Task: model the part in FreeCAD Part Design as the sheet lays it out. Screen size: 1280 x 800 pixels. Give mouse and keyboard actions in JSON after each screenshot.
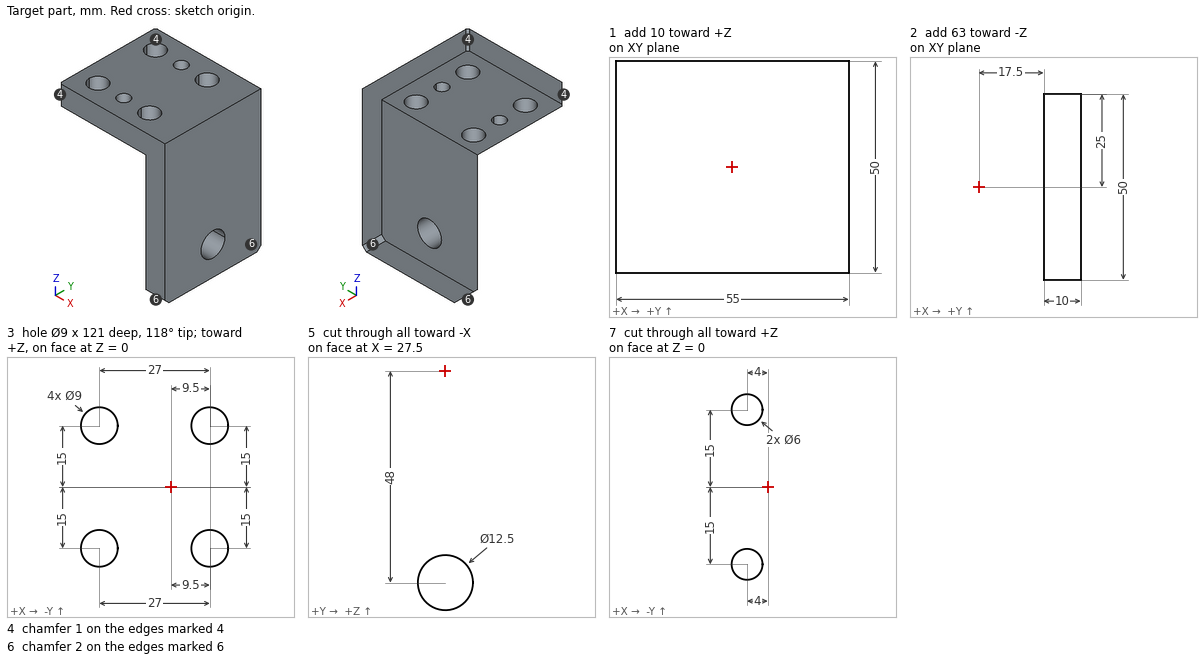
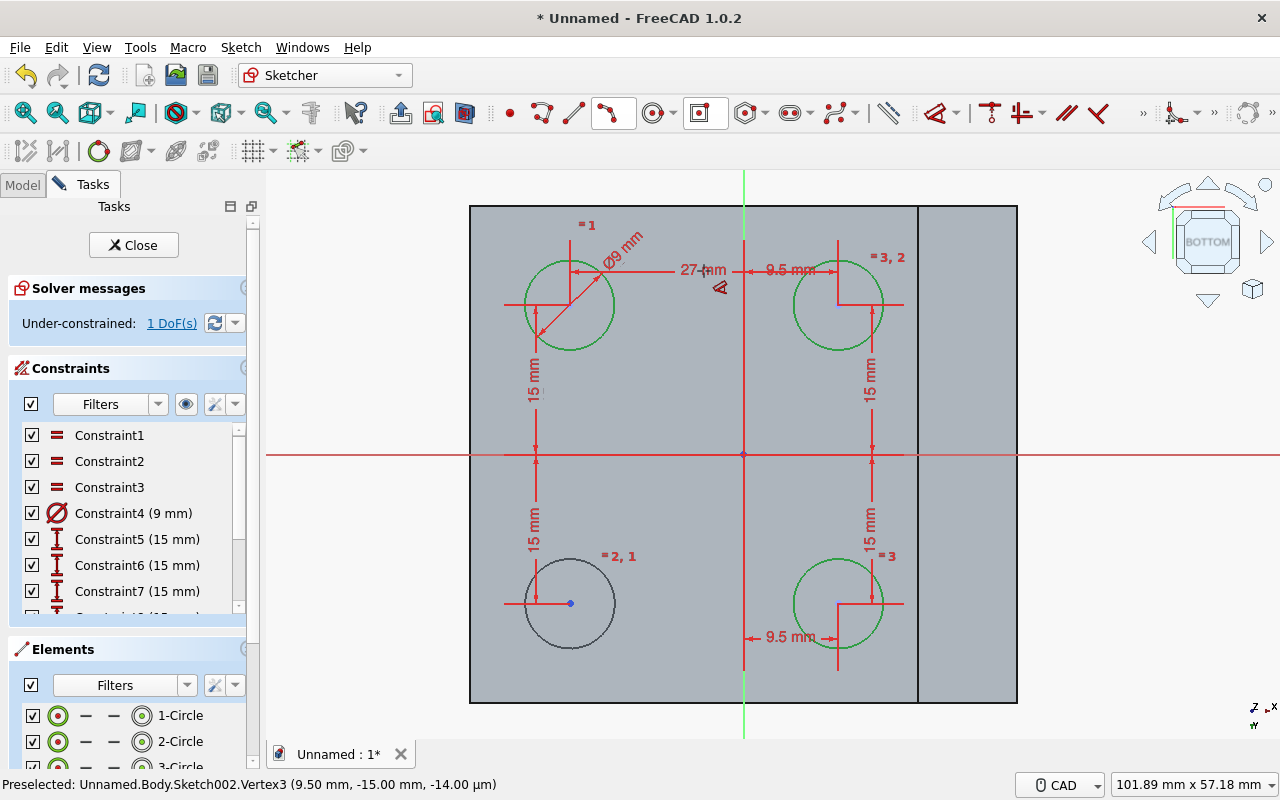
{"action": "left_click", "coordinate": [570, 604]}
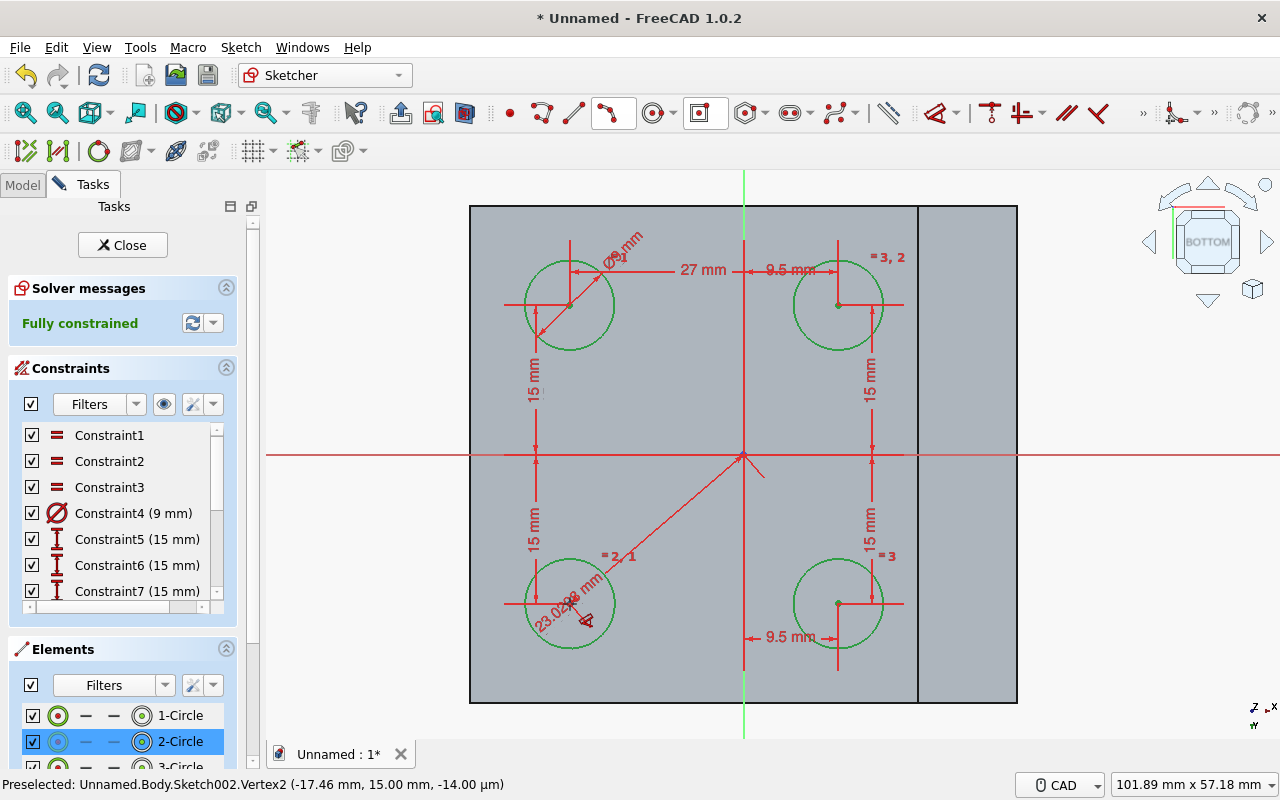
{"action": "left_click", "coordinate": [838, 305]}
{"action": "left_click", "coordinate": [704, 638]}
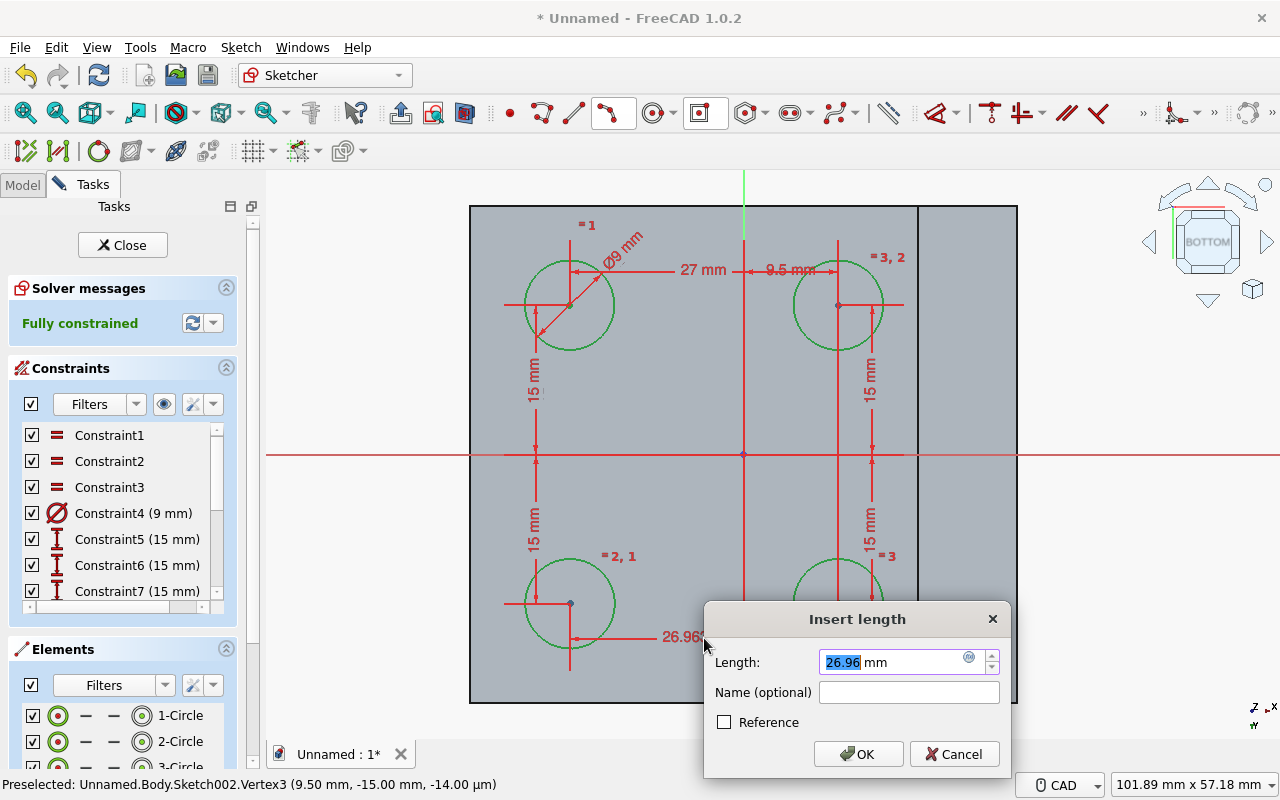
{"action": "type", "text": "27"}
{"action": "key", "text": "Return"}
{"action": "key", "text": "Escape"}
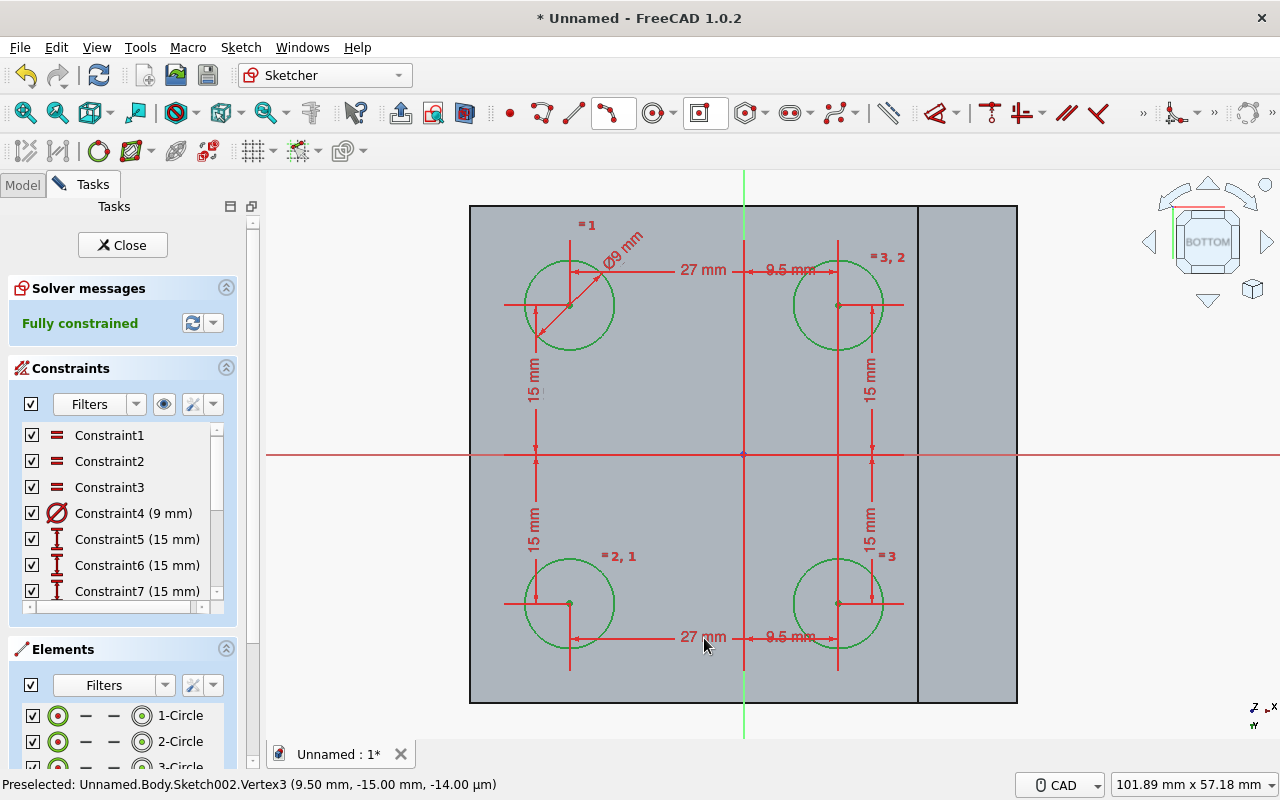
{"action": "left_click", "coordinate": [123, 245]}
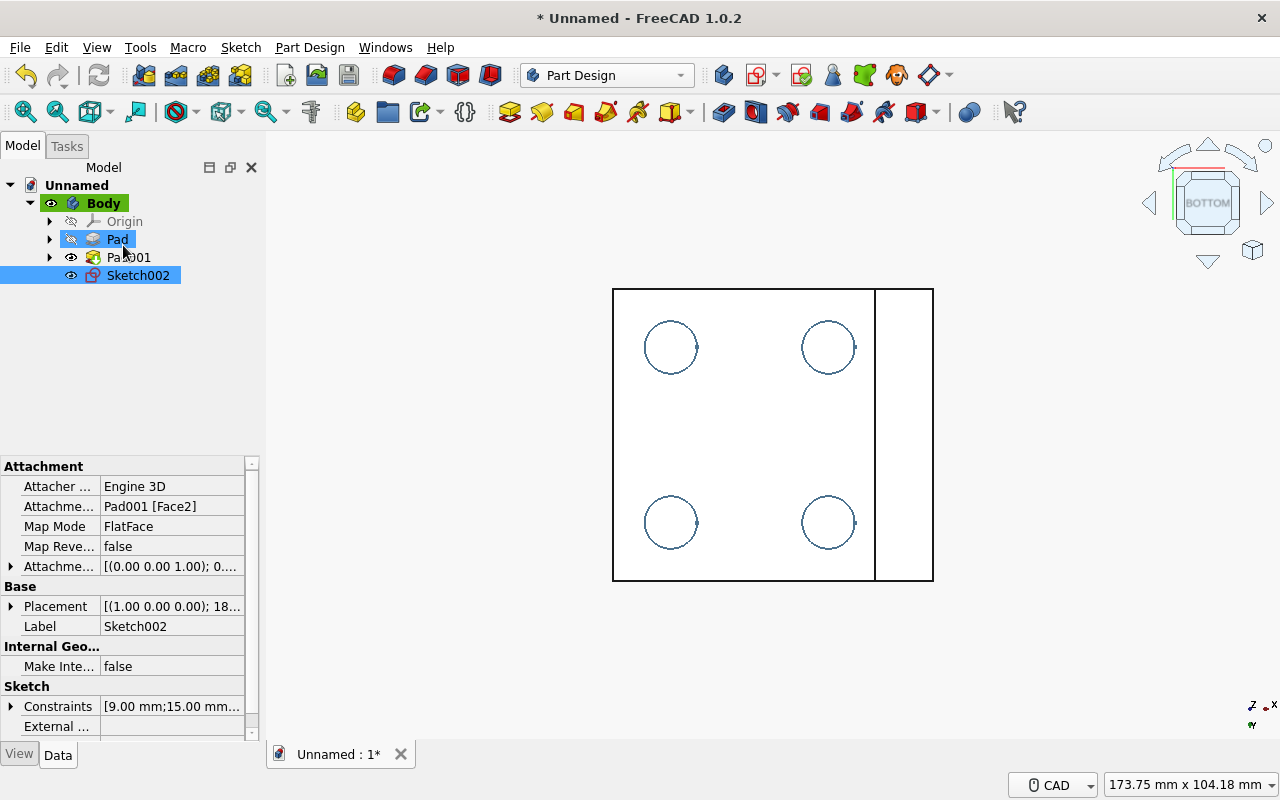
{"action": "left_click", "coordinate": [756, 112]}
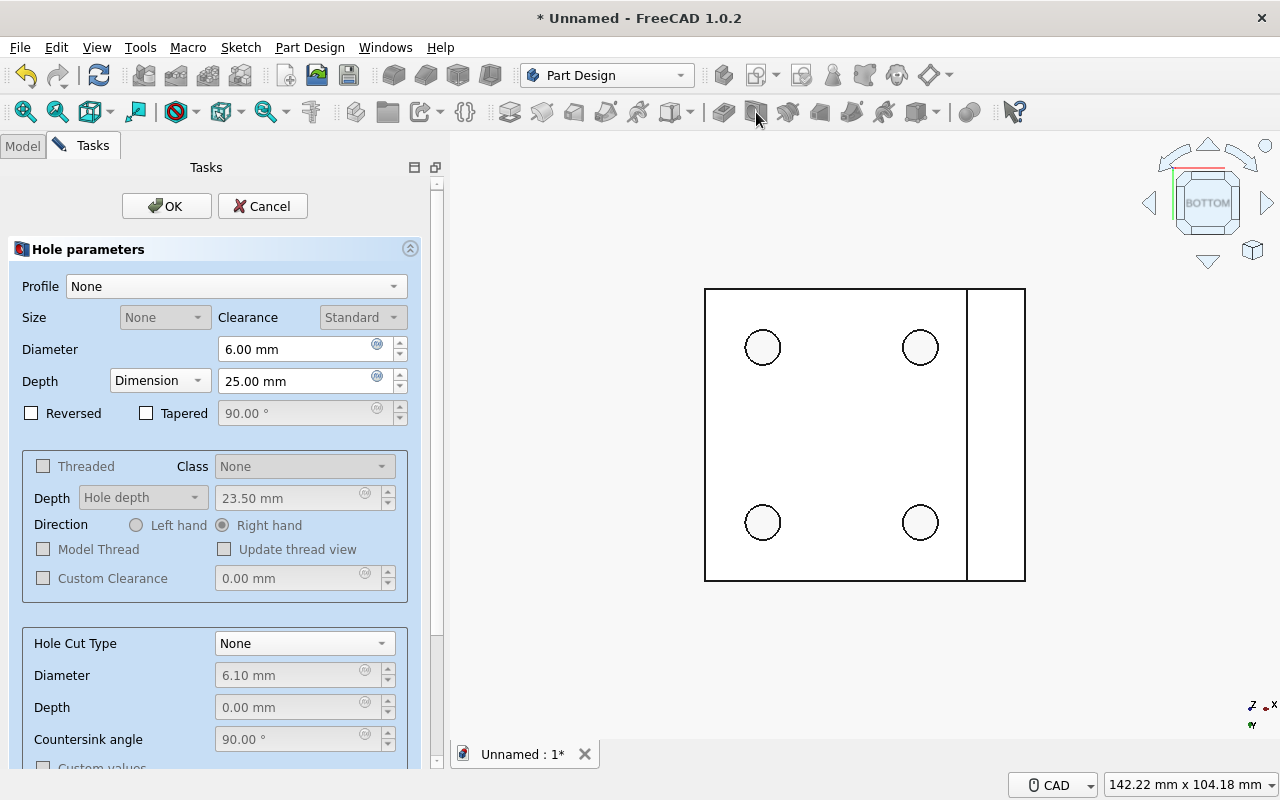
{"action": "triple_click", "coordinate": [305, 349]}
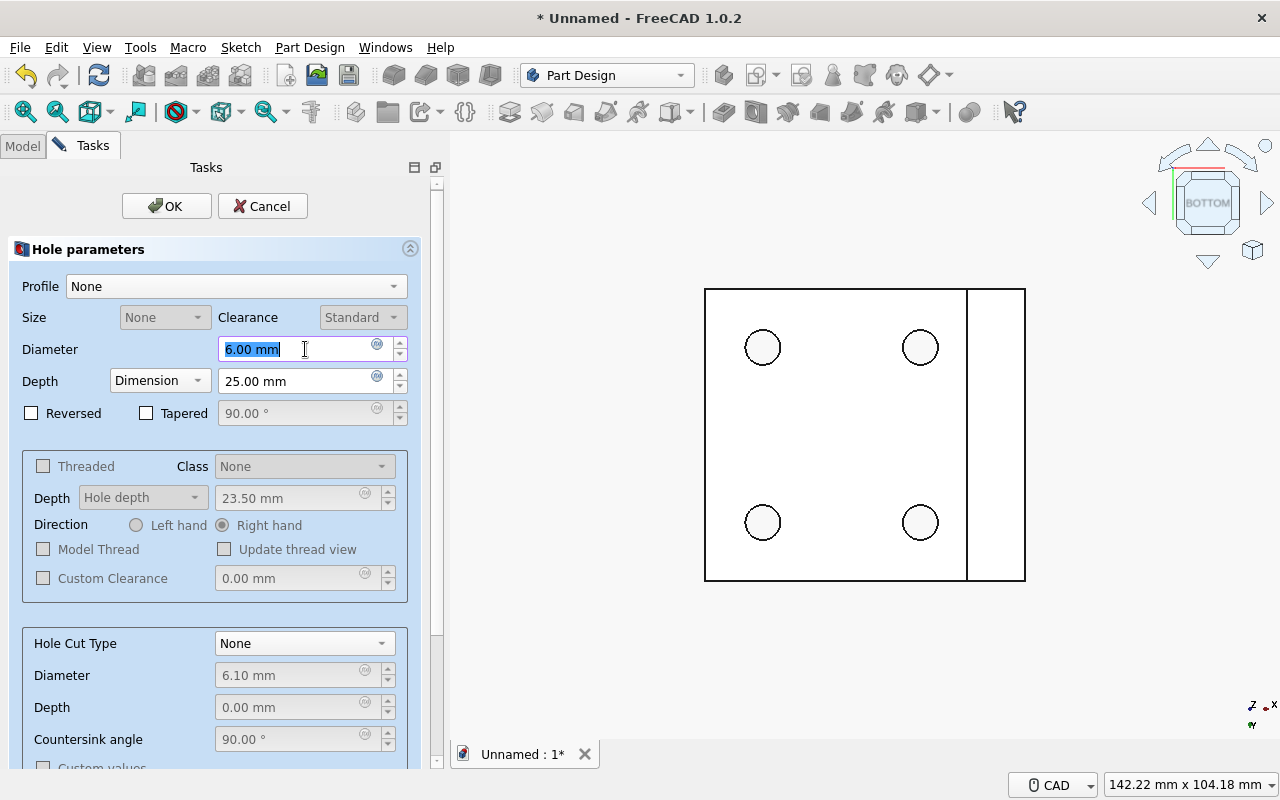
{"action": "type", "text": "9"}
{"action": "key", "text": "Tab"}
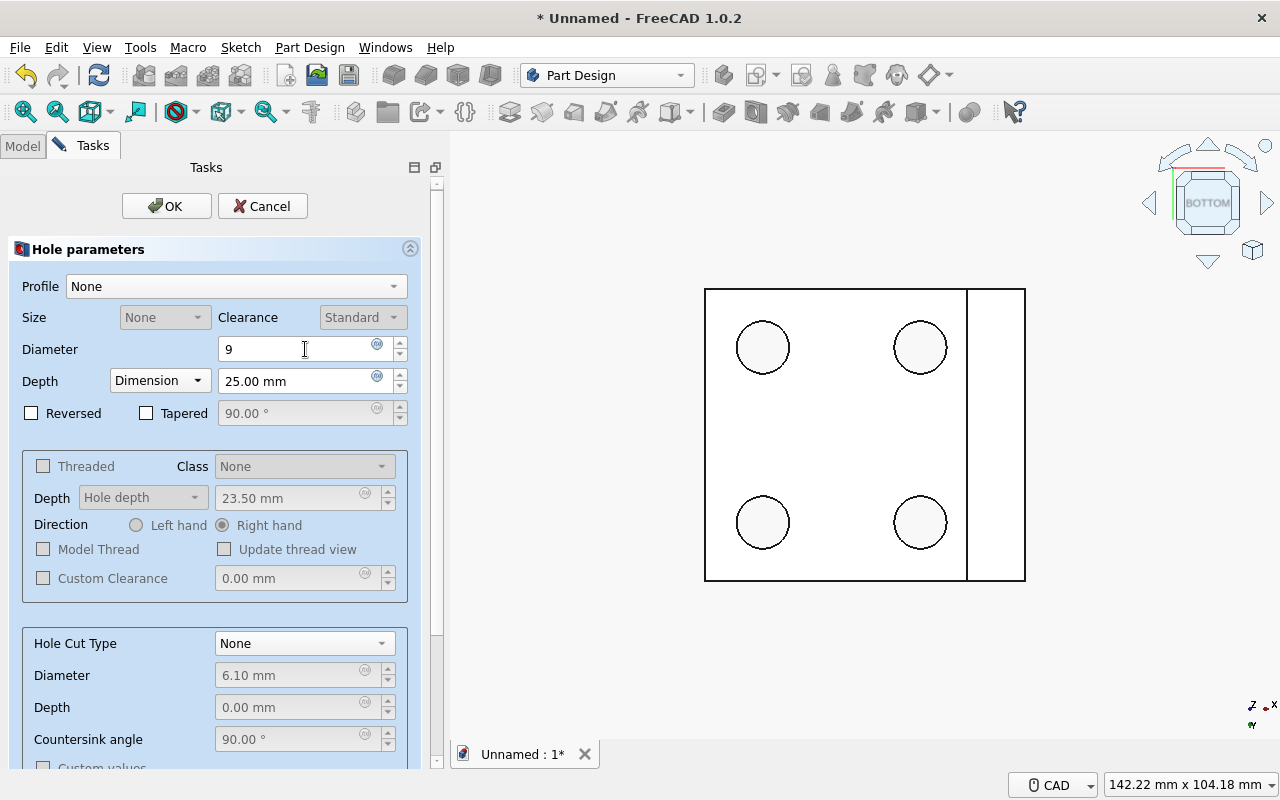
{"action": "triple_click", "coordinate": [305, 381]}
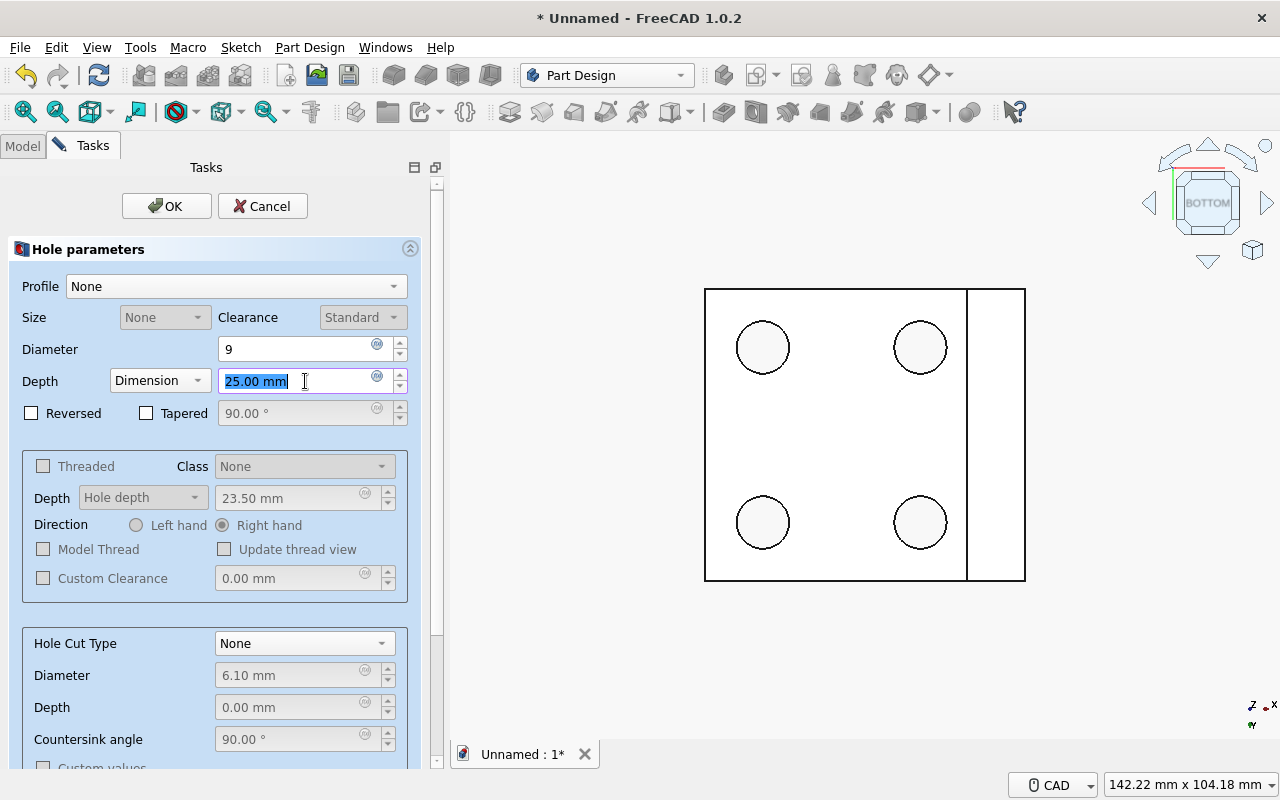
{"action": "type", "text": "121"}
{"action": "key", "text": "Tab"}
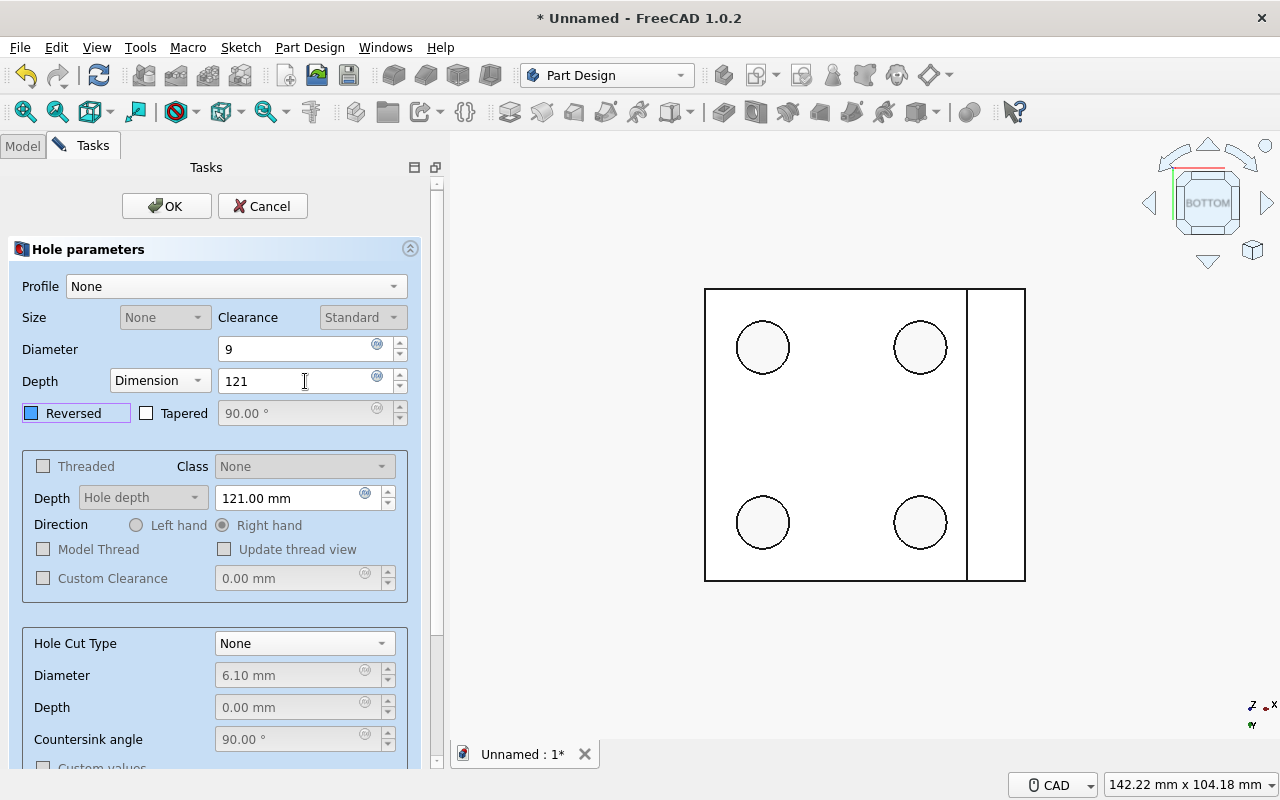
{"action": "left_click", "coordinate": [167, 206]}